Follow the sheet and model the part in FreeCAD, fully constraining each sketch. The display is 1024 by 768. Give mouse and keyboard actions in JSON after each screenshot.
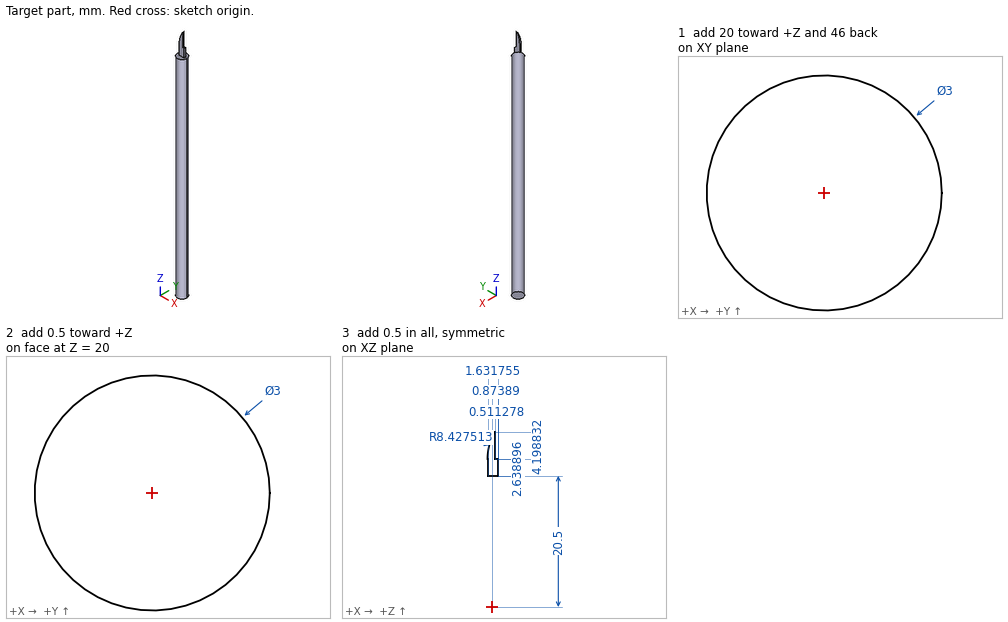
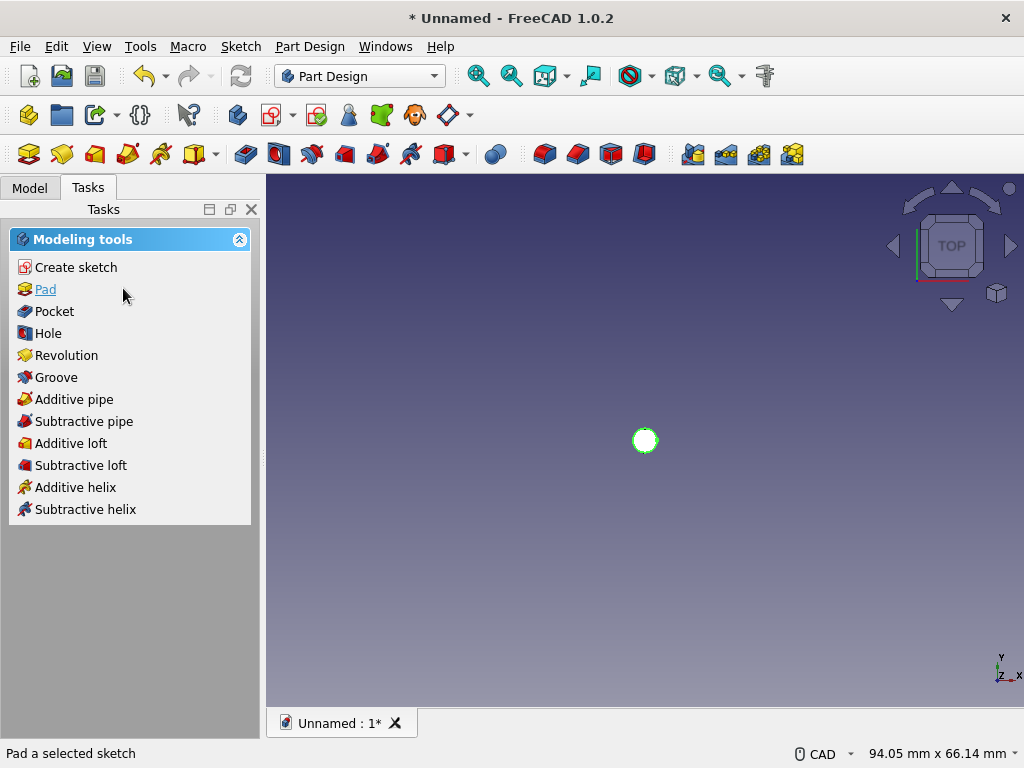
{"action": "left_click", "coordinate": [29, 154]}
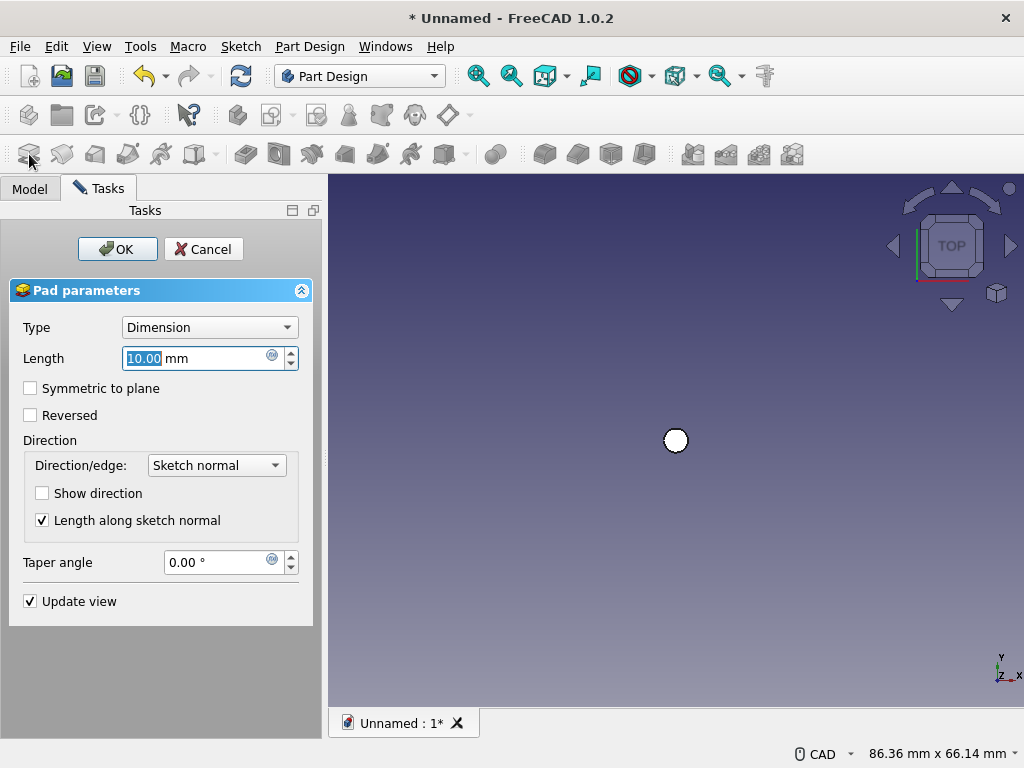
{"action": "type", "text": "0.5"}
{"action": "key", "text": "Tab"}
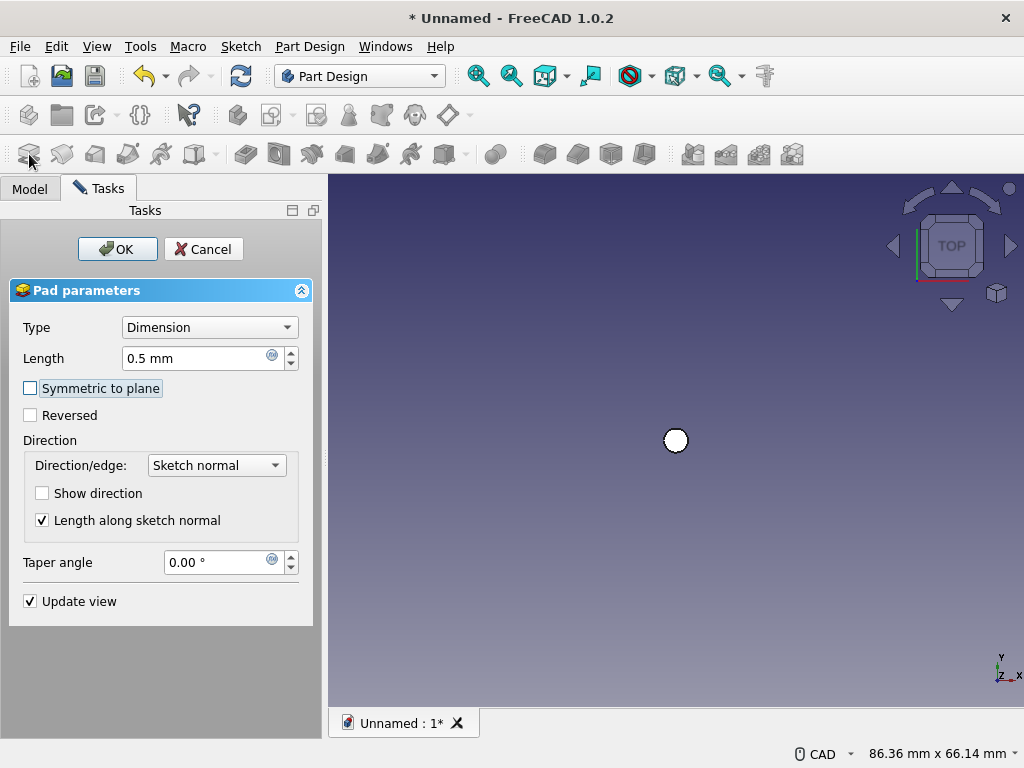
{"action": "left_click", "coordinate": [118, 249]}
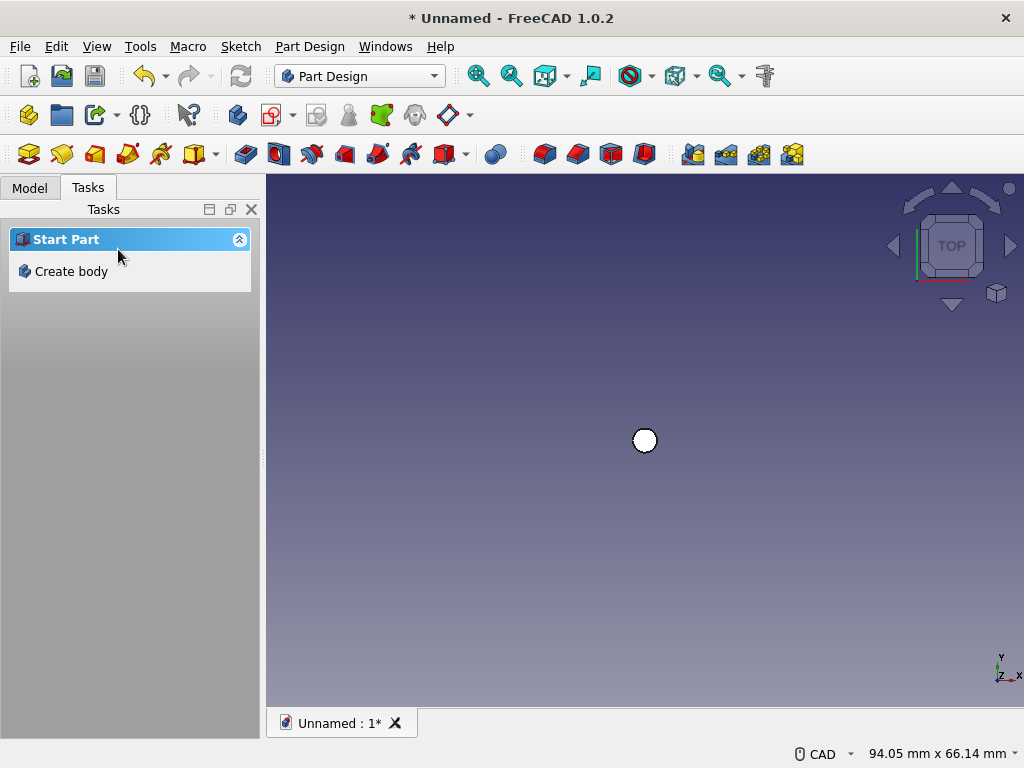
{"action": "left_click", "coordinate": [479, 76]}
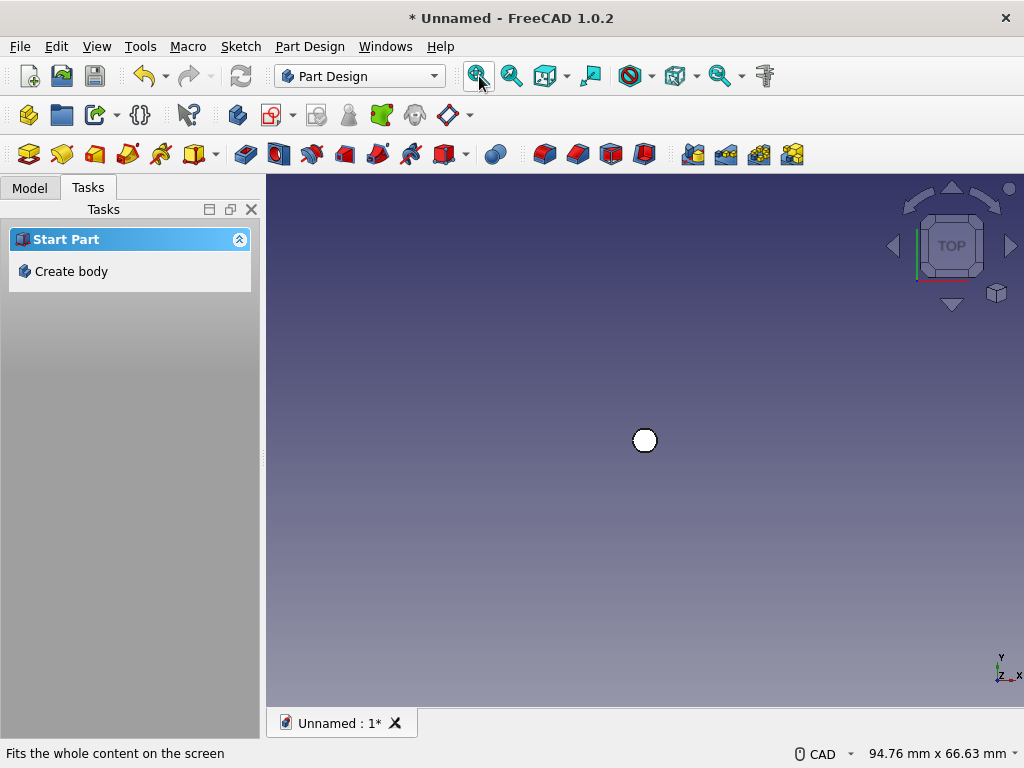
{"action": "left_click", "coordinate": [270, 116]}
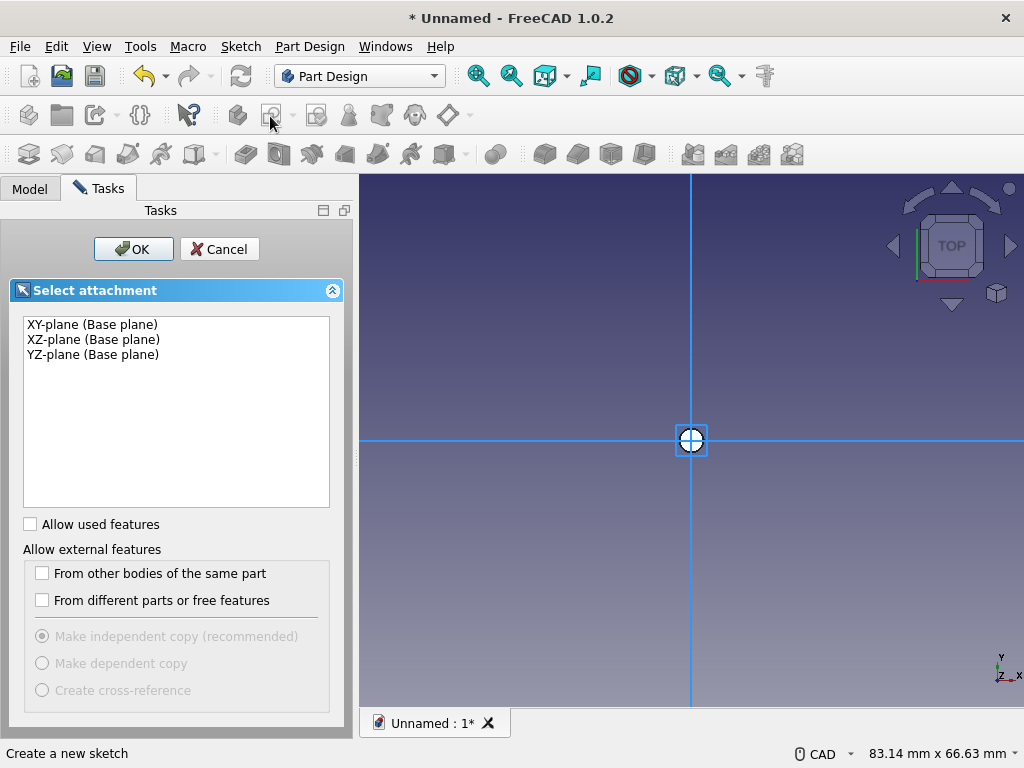
{"action": "left_click", "coordinate": [84, 340]}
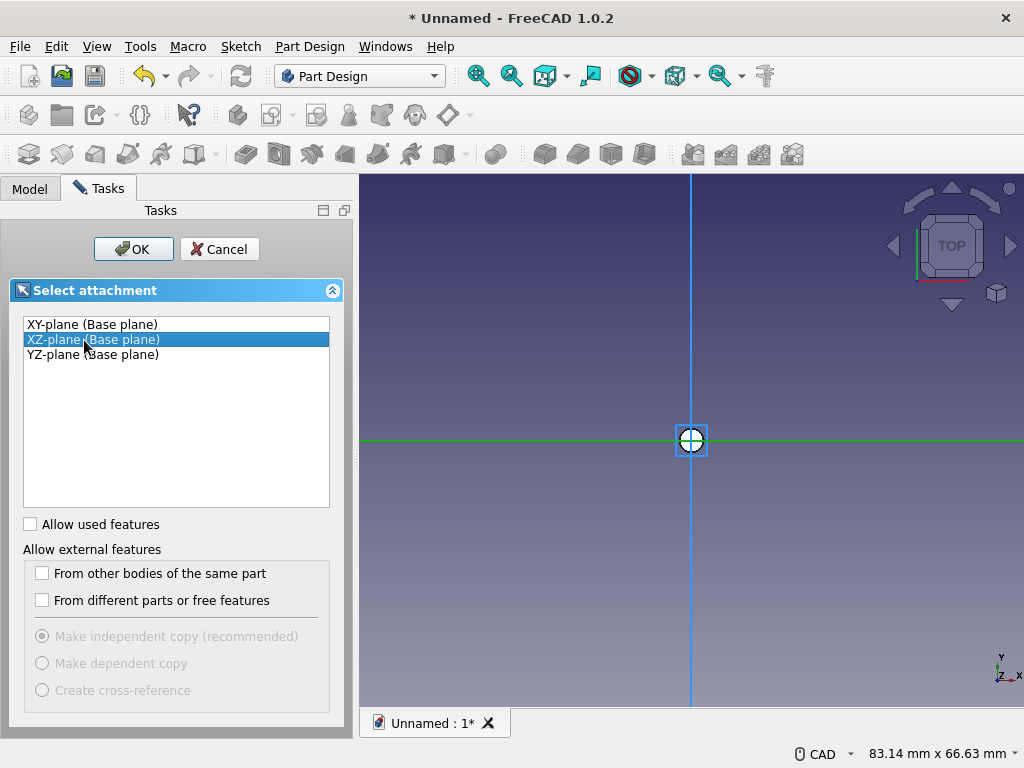
{"action": "left_click", "coordinate": [134, 249]}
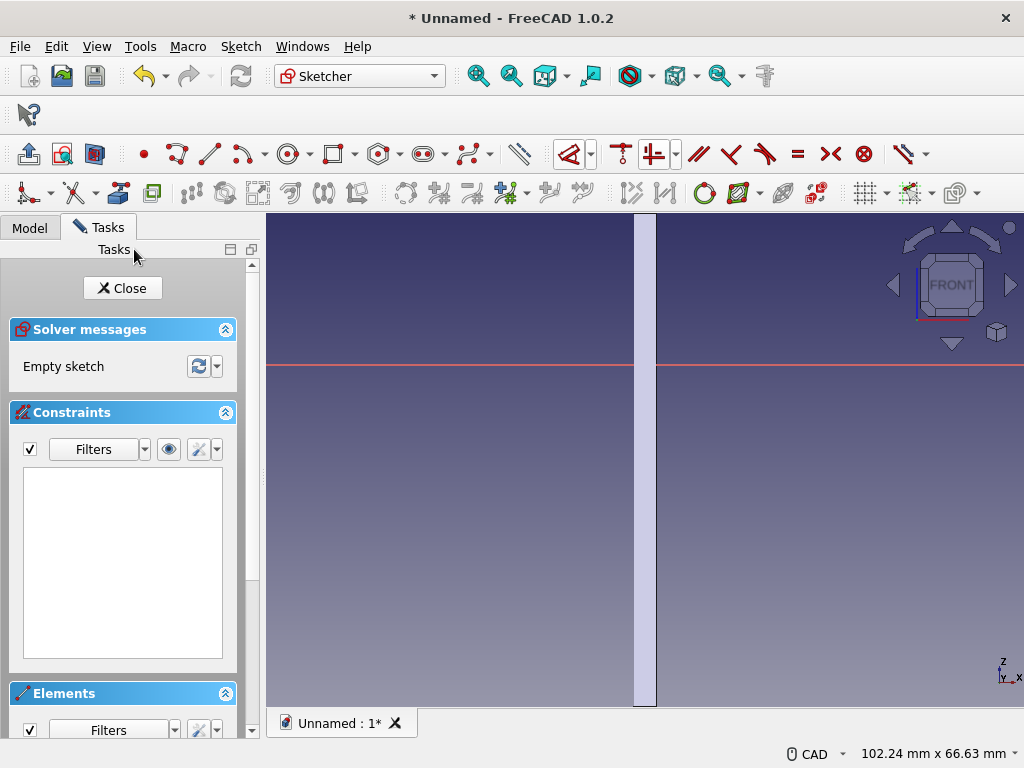
{"action": "left_click", "coordinate": [95, 154]}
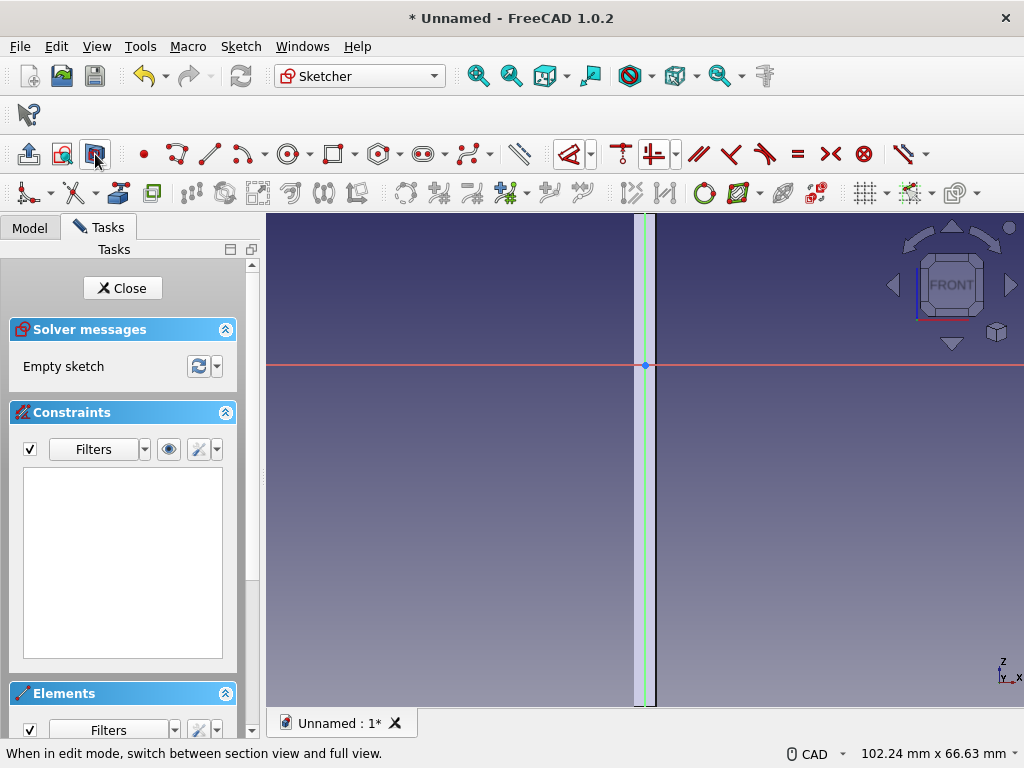
{"action": "scroll", "coordinate": [576, 460], "scroll_direction": "down", "scroll_amount": 5}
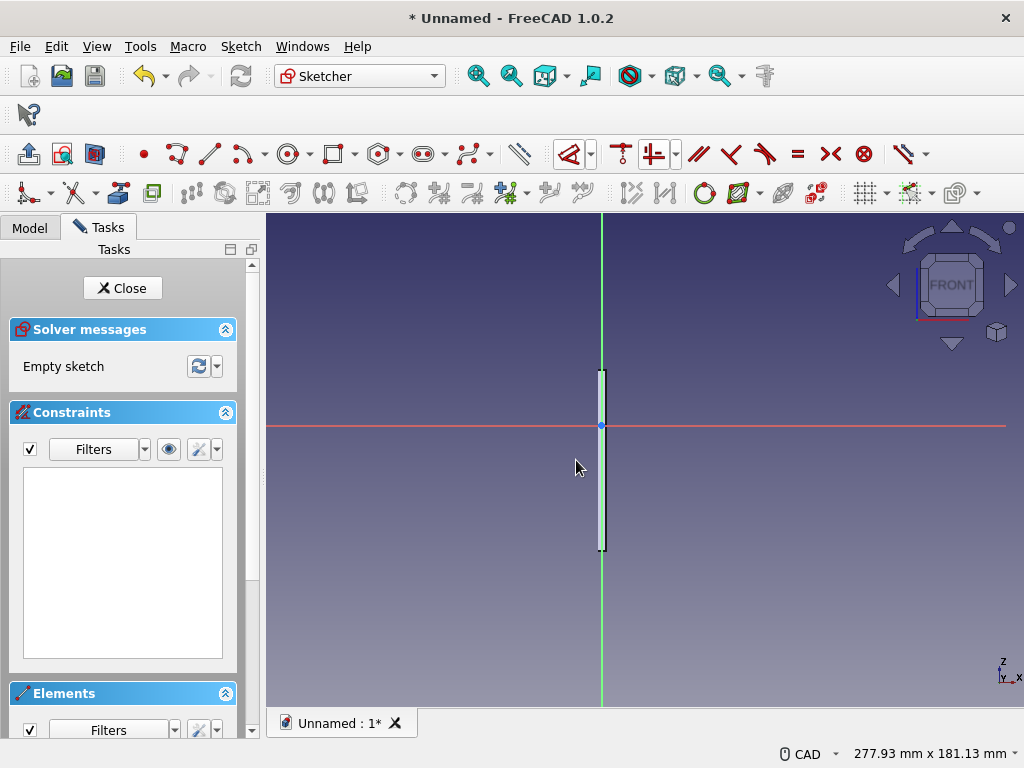
{"action": "scroll", "coordinate": [603, 354], "scroll_direction": "up", "scroll_amount": 14}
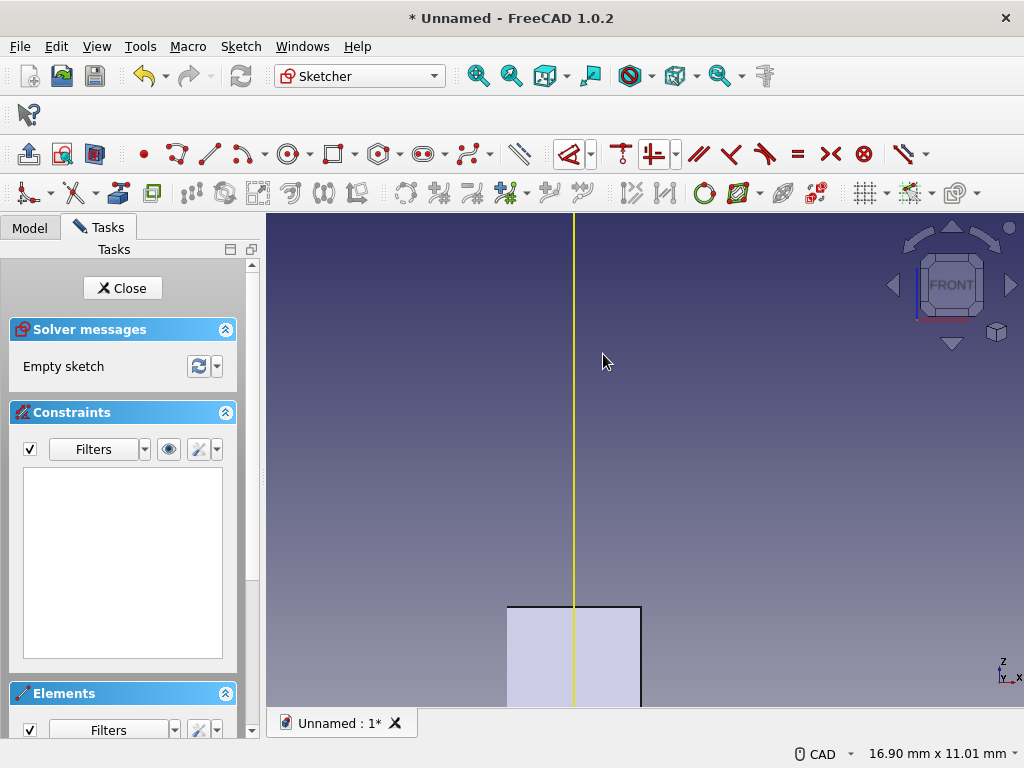
{"action": "left_click", "coordinate": [177, 154]}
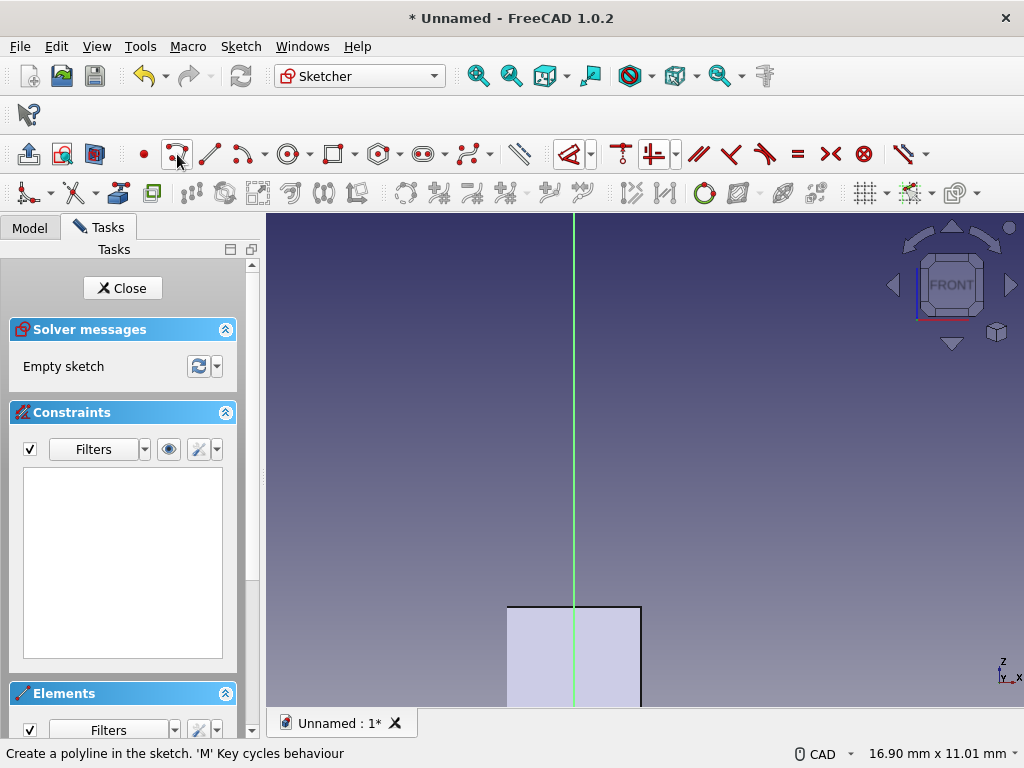
{"action": "left_click", "coordinate": [590, 300]}
{"action": "left_click", "coordinate": [590, 488]}
{"action": "left_click", "coordinate": [613, 488]}
{"action": "left_click", "coordinate": [613, 607]}
{"action": "left_click", "coordinate": [540, 607]}
{"action": "left_click", "coordinate": [540, 488]}
{"action": "right_click", "coordinate": [540, 488]}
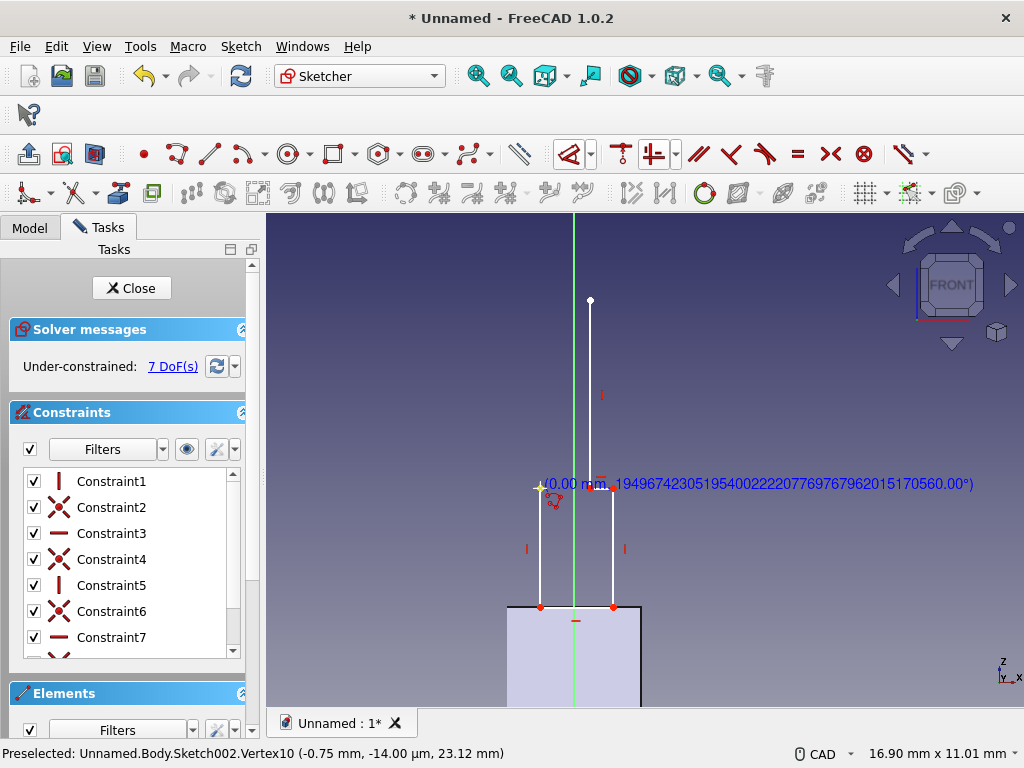
{"action": "key", "text": "g 3 a"}